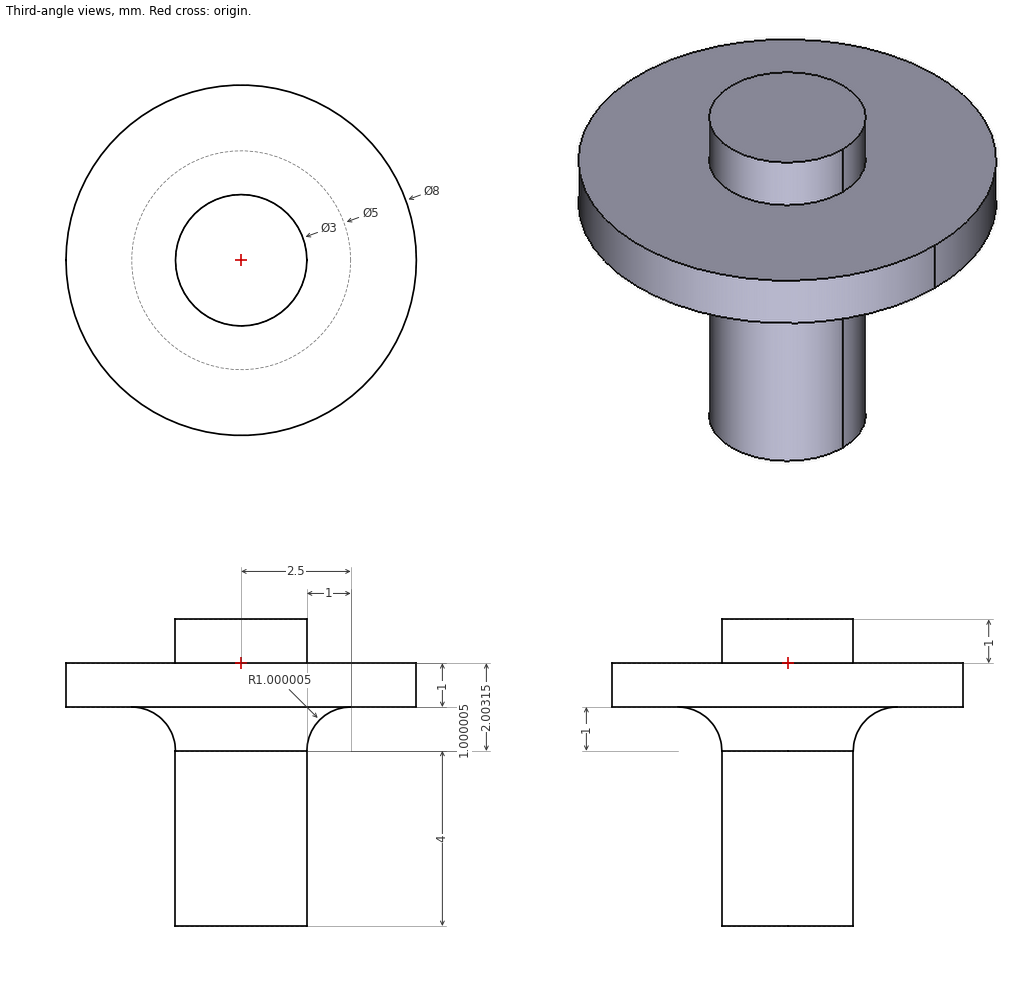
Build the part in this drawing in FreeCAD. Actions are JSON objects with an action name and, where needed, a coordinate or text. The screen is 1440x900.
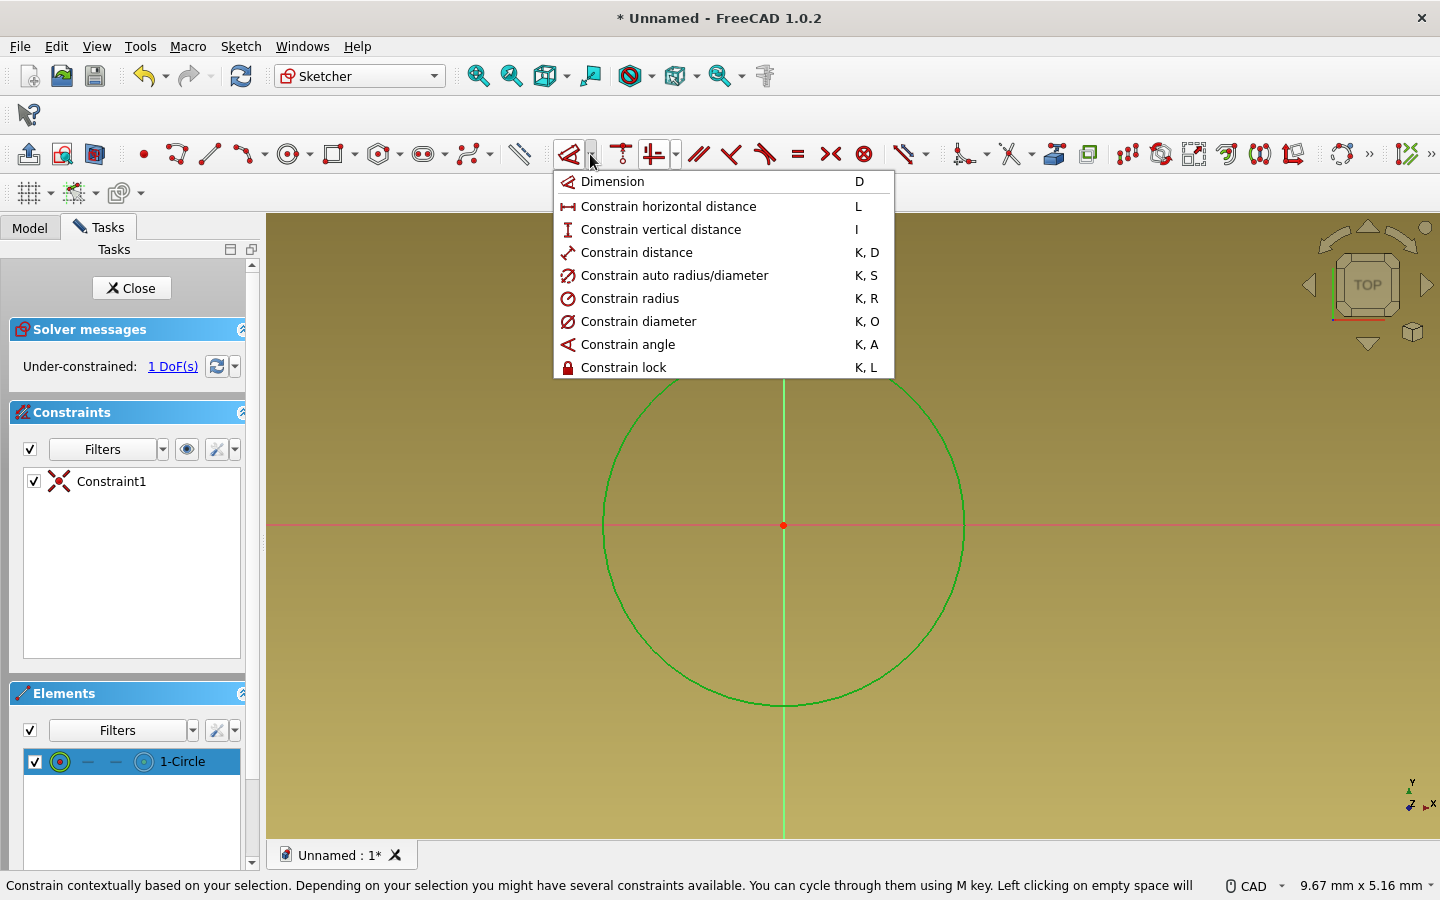
{"action": "left_click", "coordinate": [724, 322]}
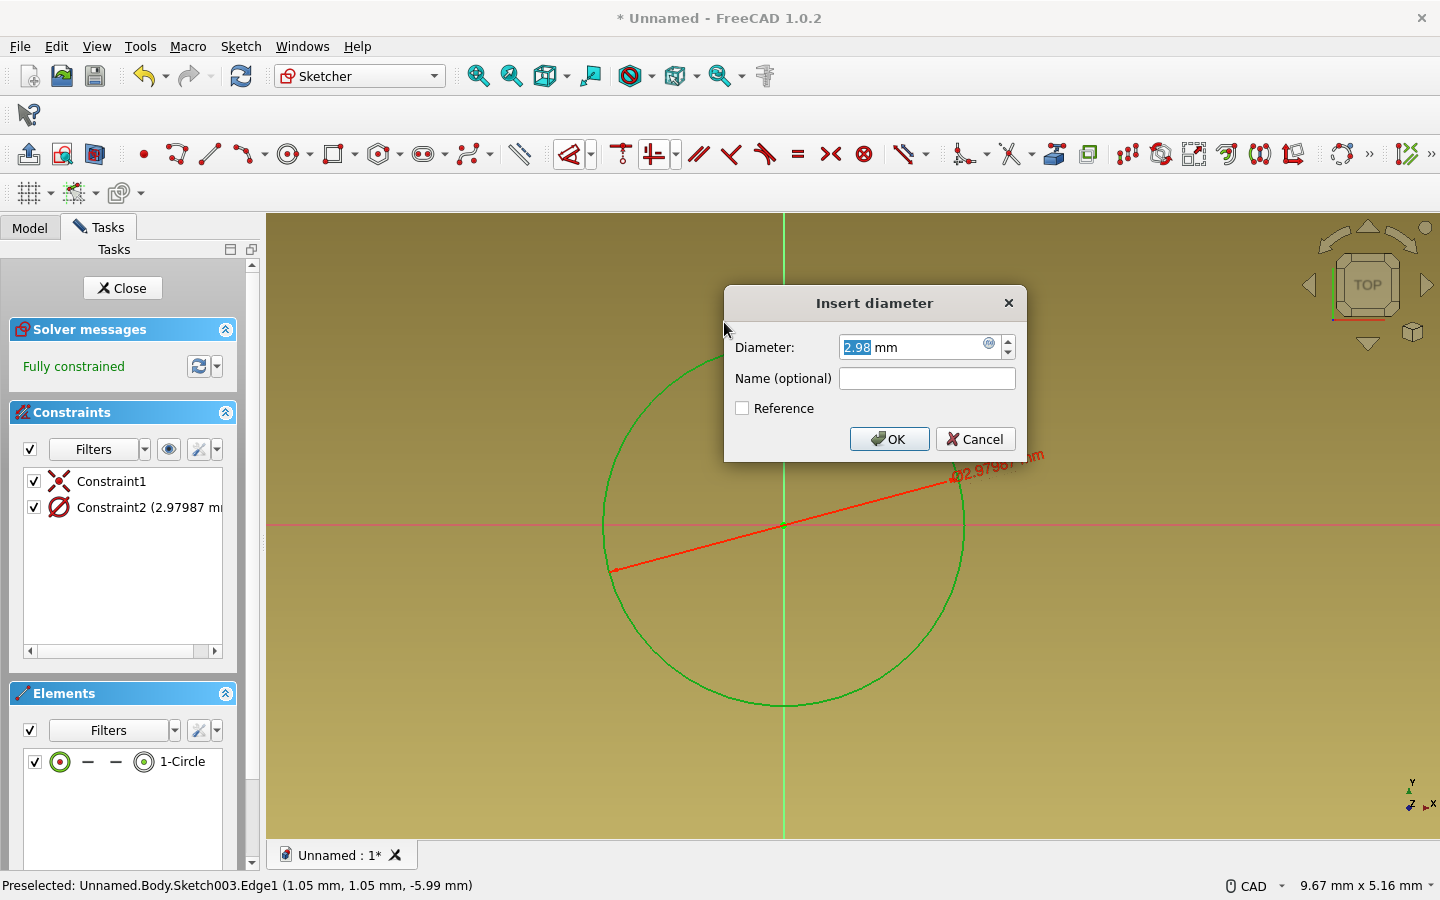
{"action": "type", "text": "3"}
{"action": "key", "text": "Return"}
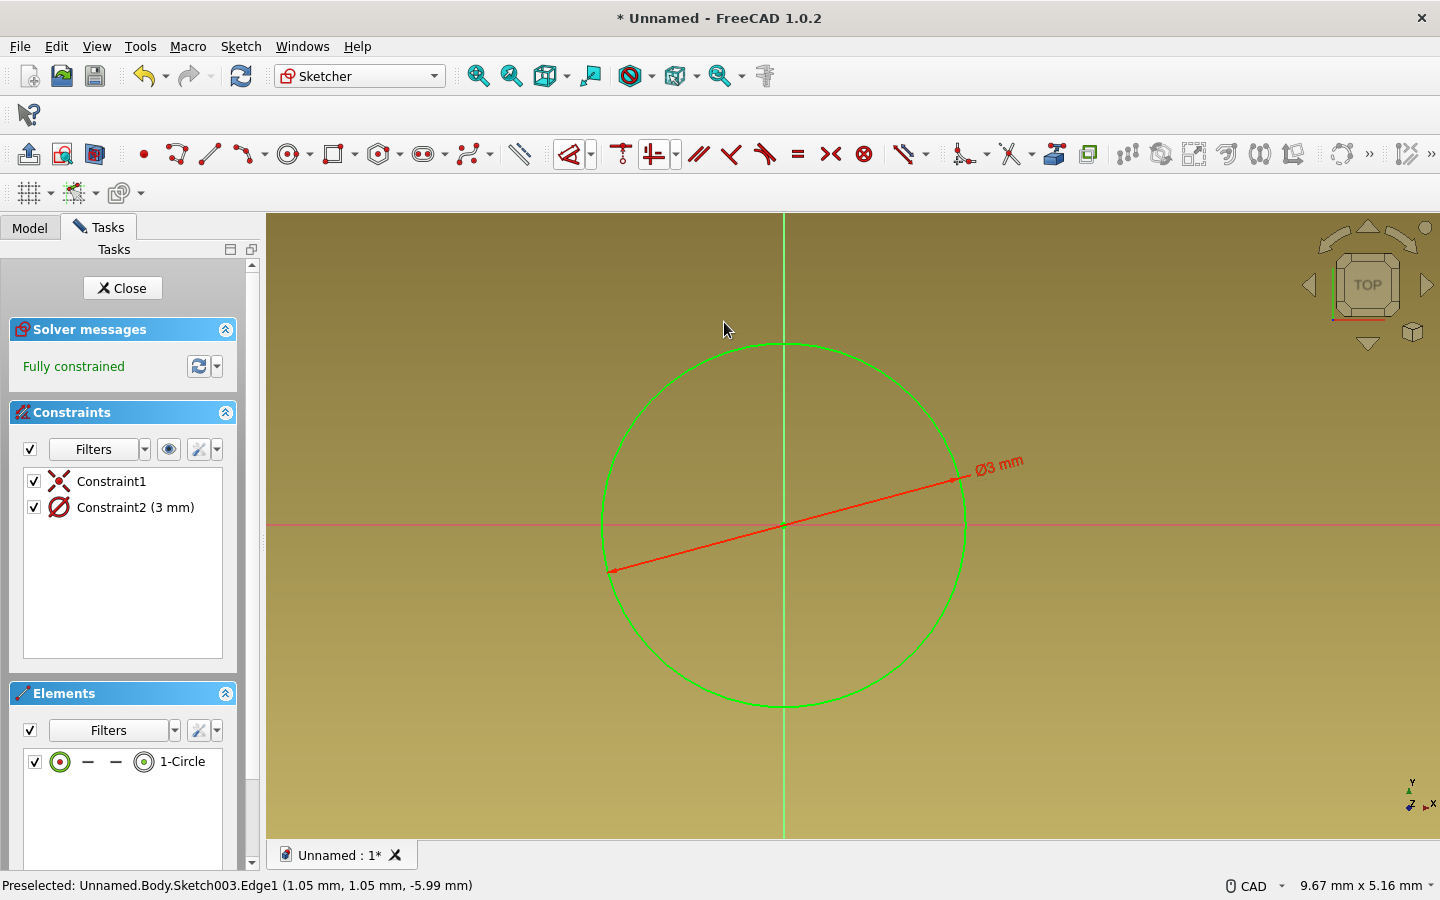
{"action": "left_click", "coordinate": [123, 288]}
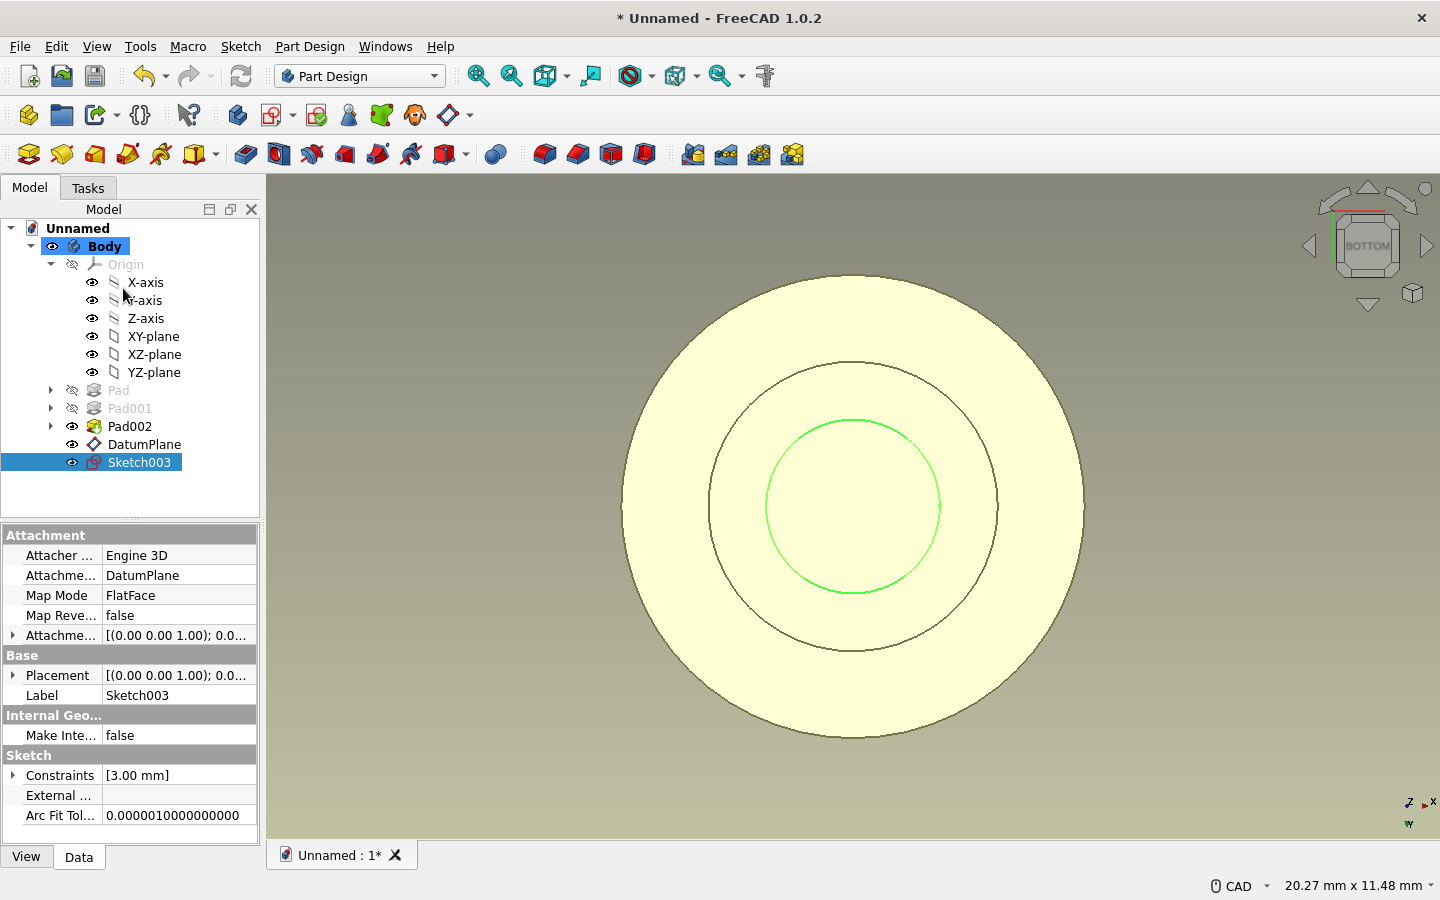
{"action": "left_click", "coordinate": [29, 154]}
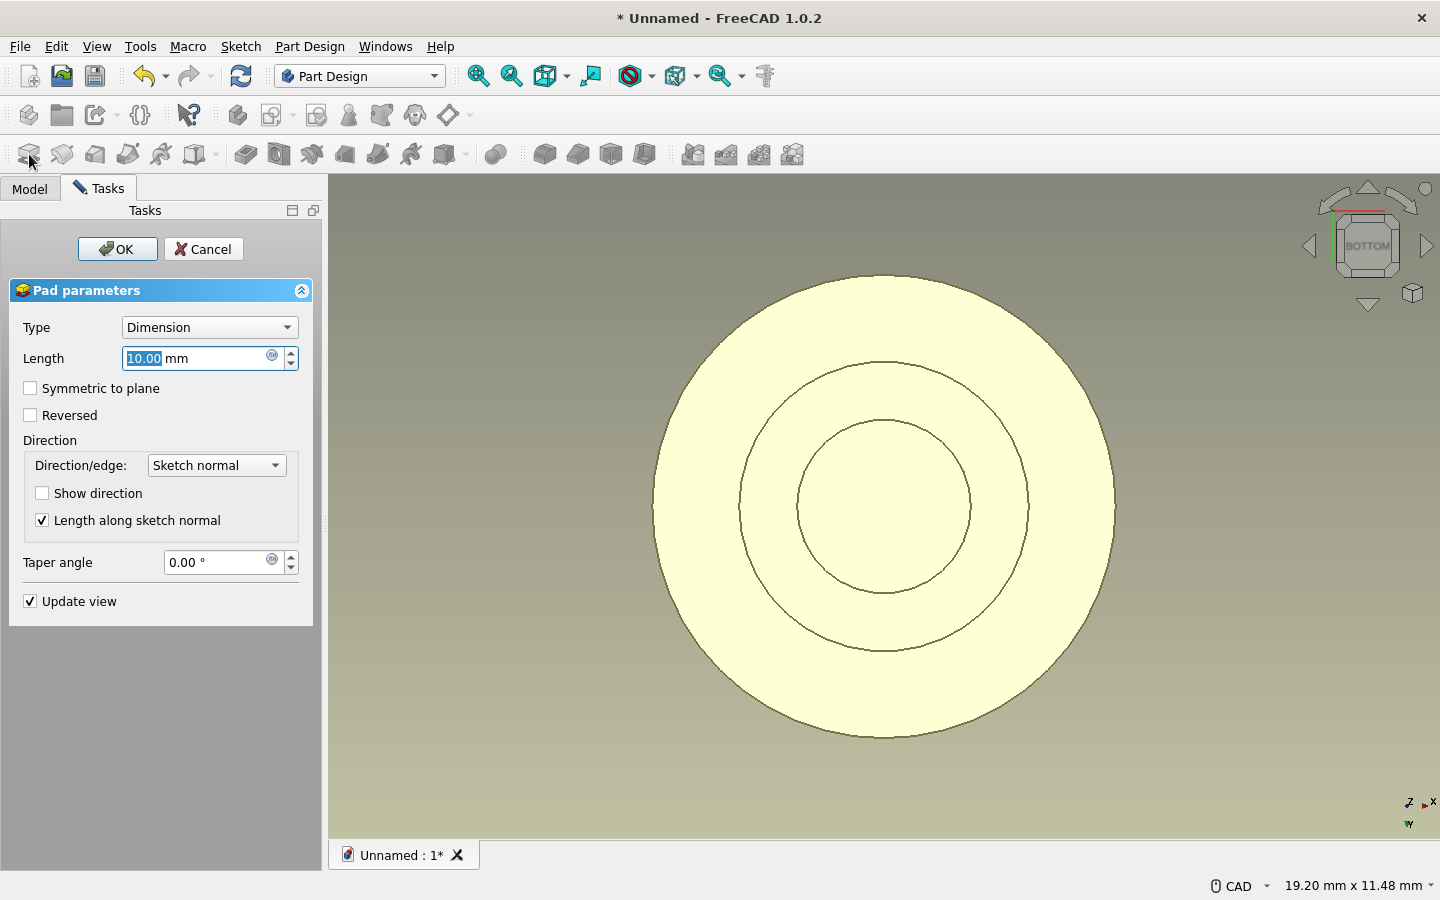
{"action": "type", "text": "4"}
{"action": "key", "text": "Tab"}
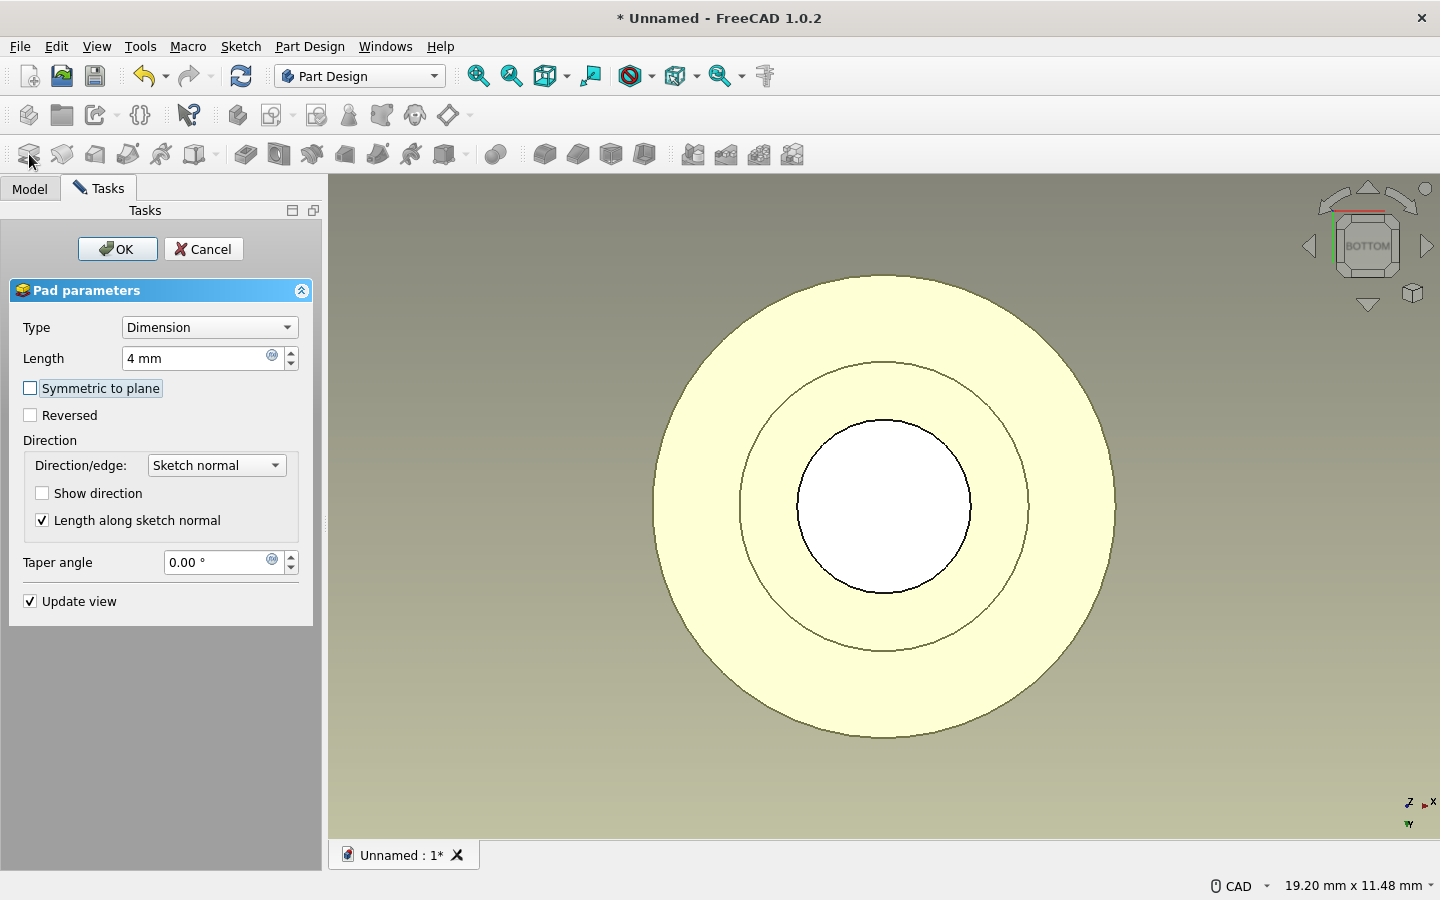
{"action": "left_click", "coordinate": [118, 249]}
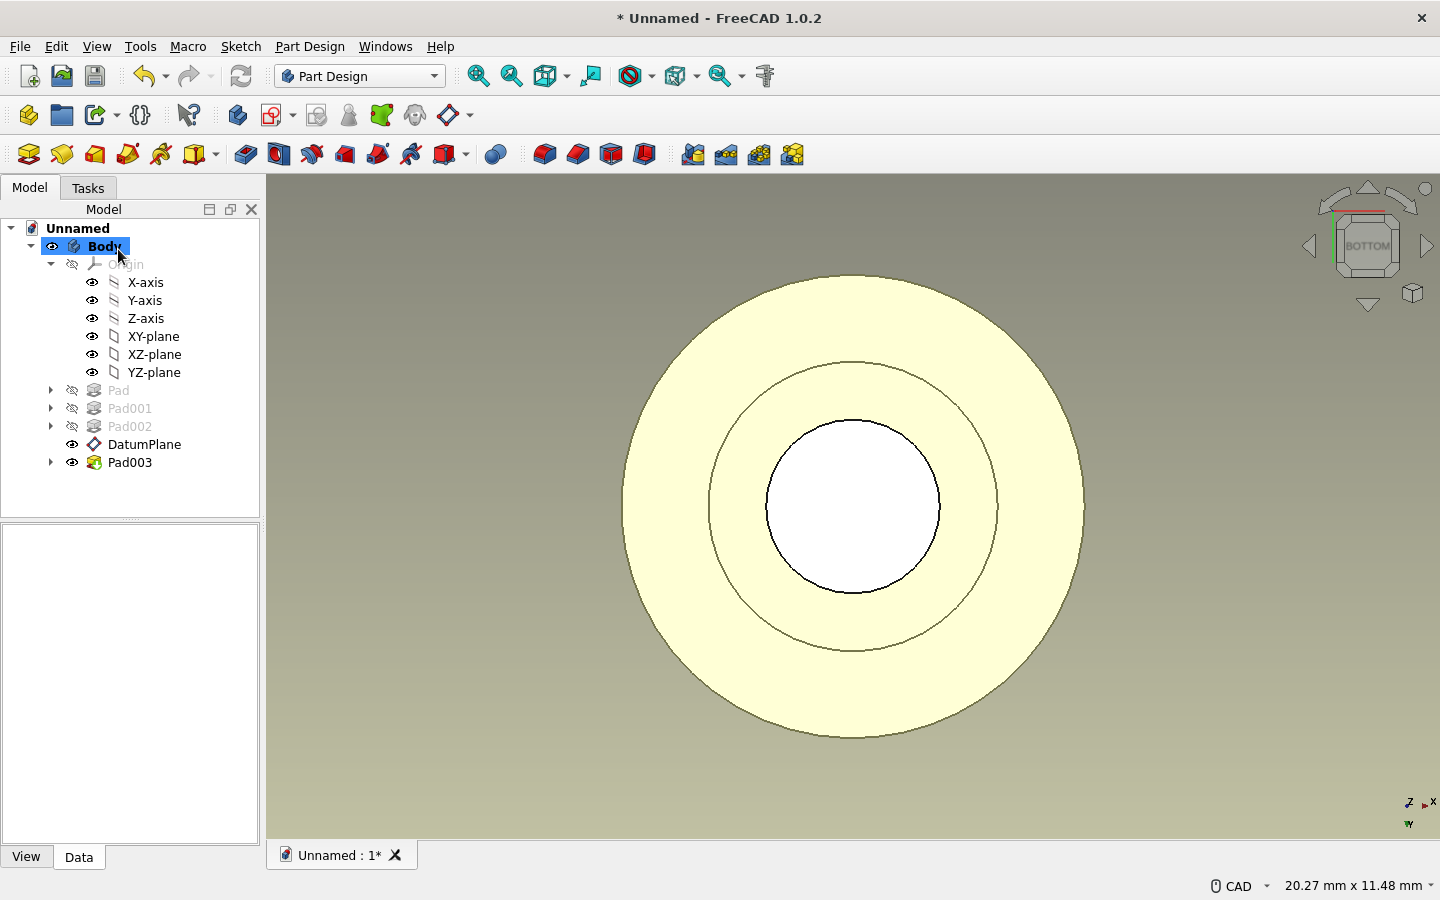
{"action": "left_click", "coordinate": [117, 444]}
{"action": "key", "text": "space"}